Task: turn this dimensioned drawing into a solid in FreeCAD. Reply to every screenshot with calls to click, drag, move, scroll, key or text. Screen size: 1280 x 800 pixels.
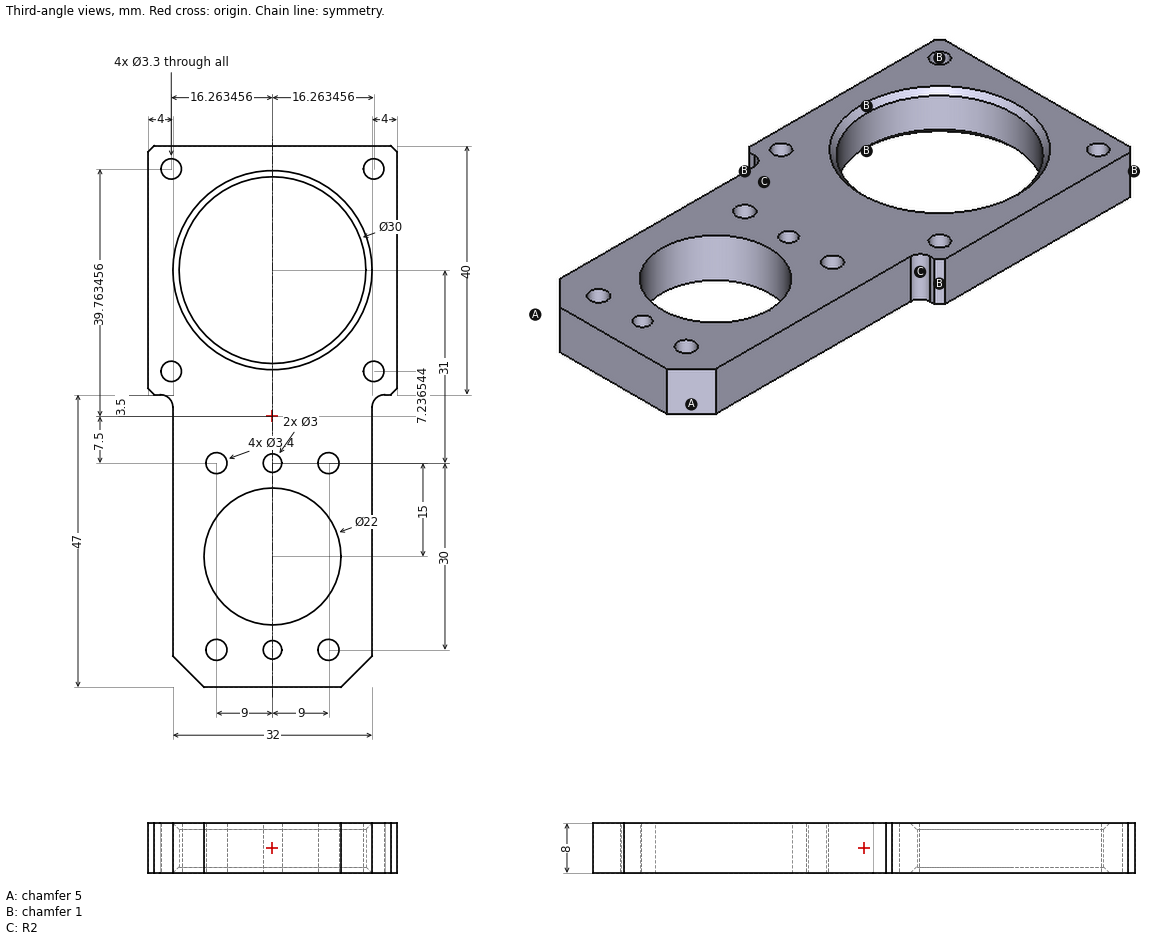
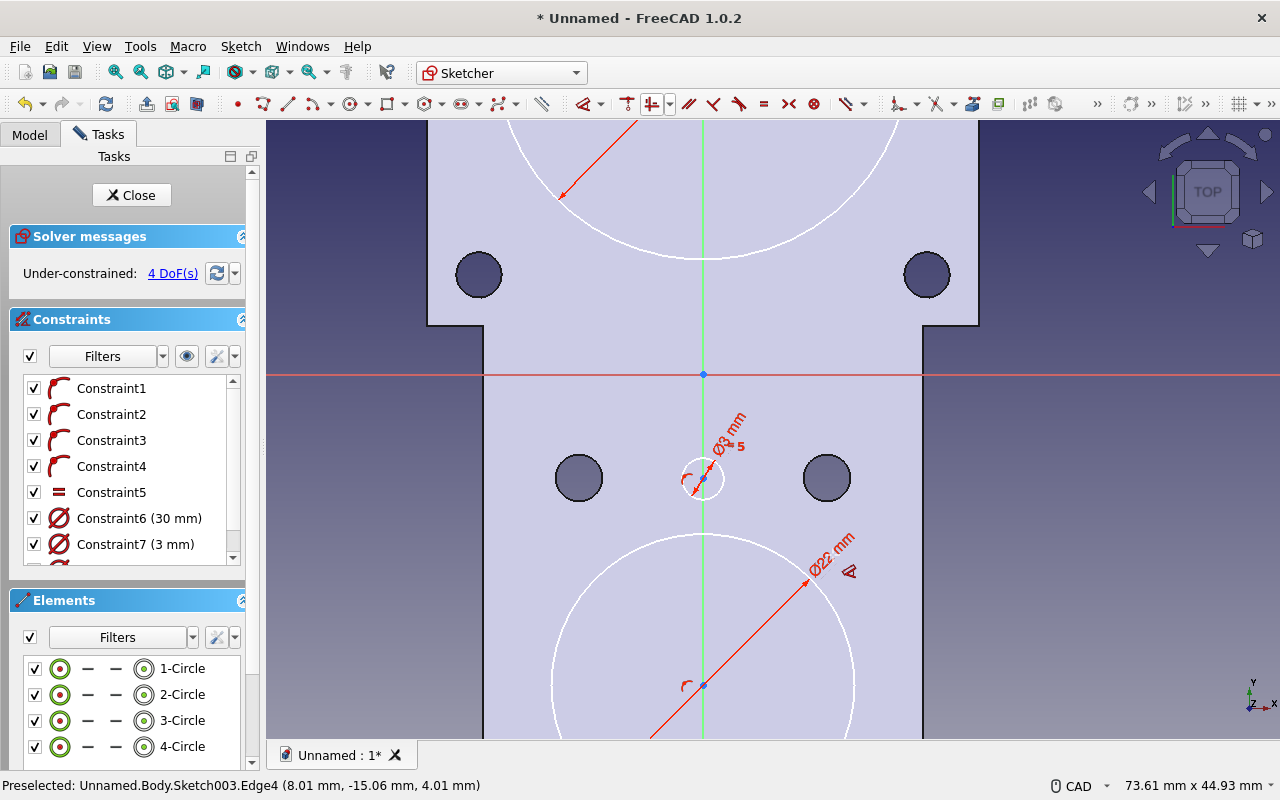
click(703, 479)
click(737, 403)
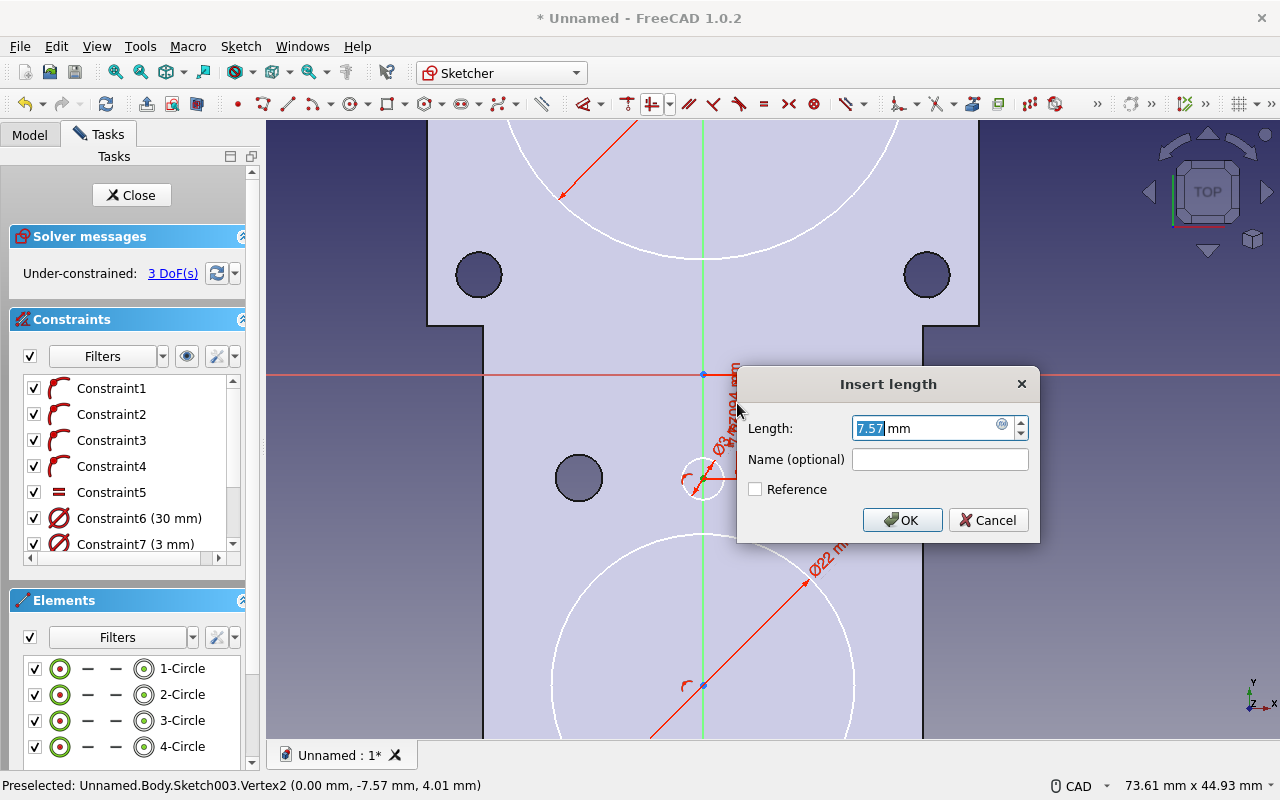
text(7.5)
key(Return)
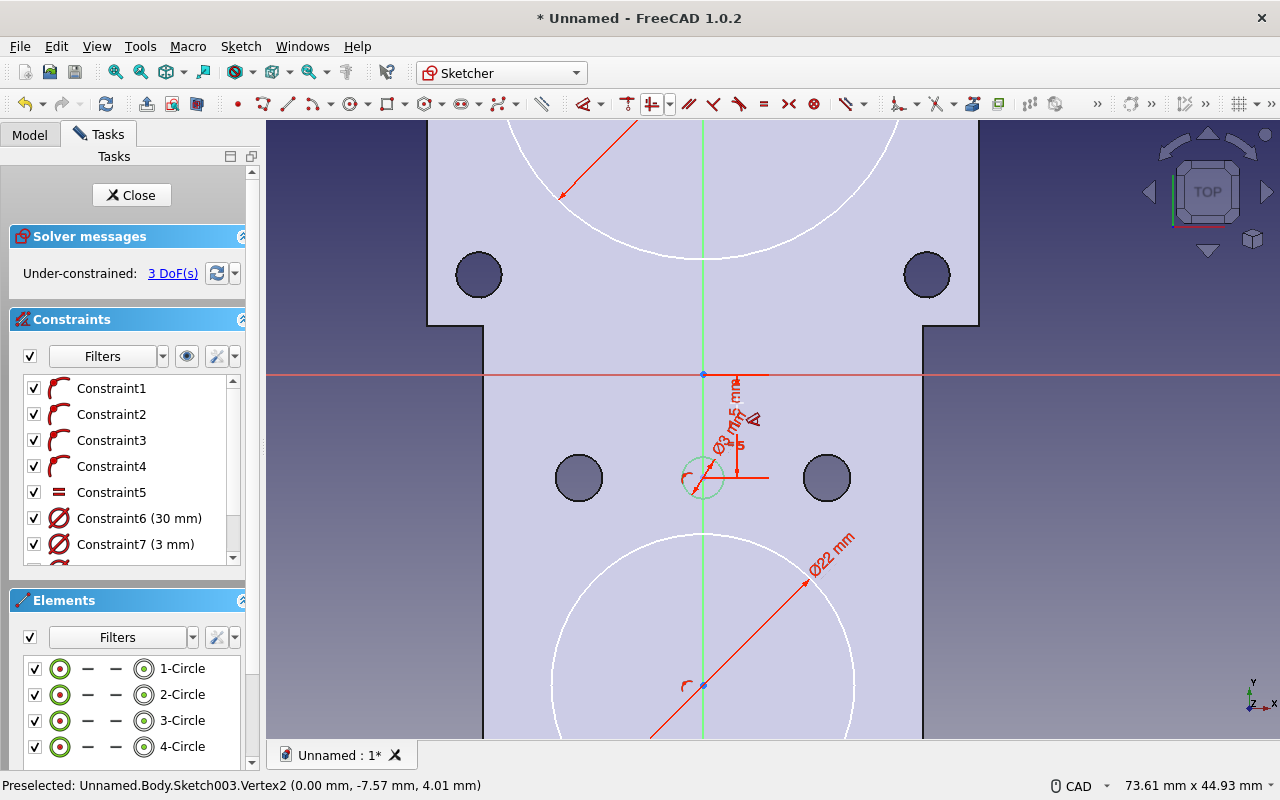
scroll(705, 459, down, 5)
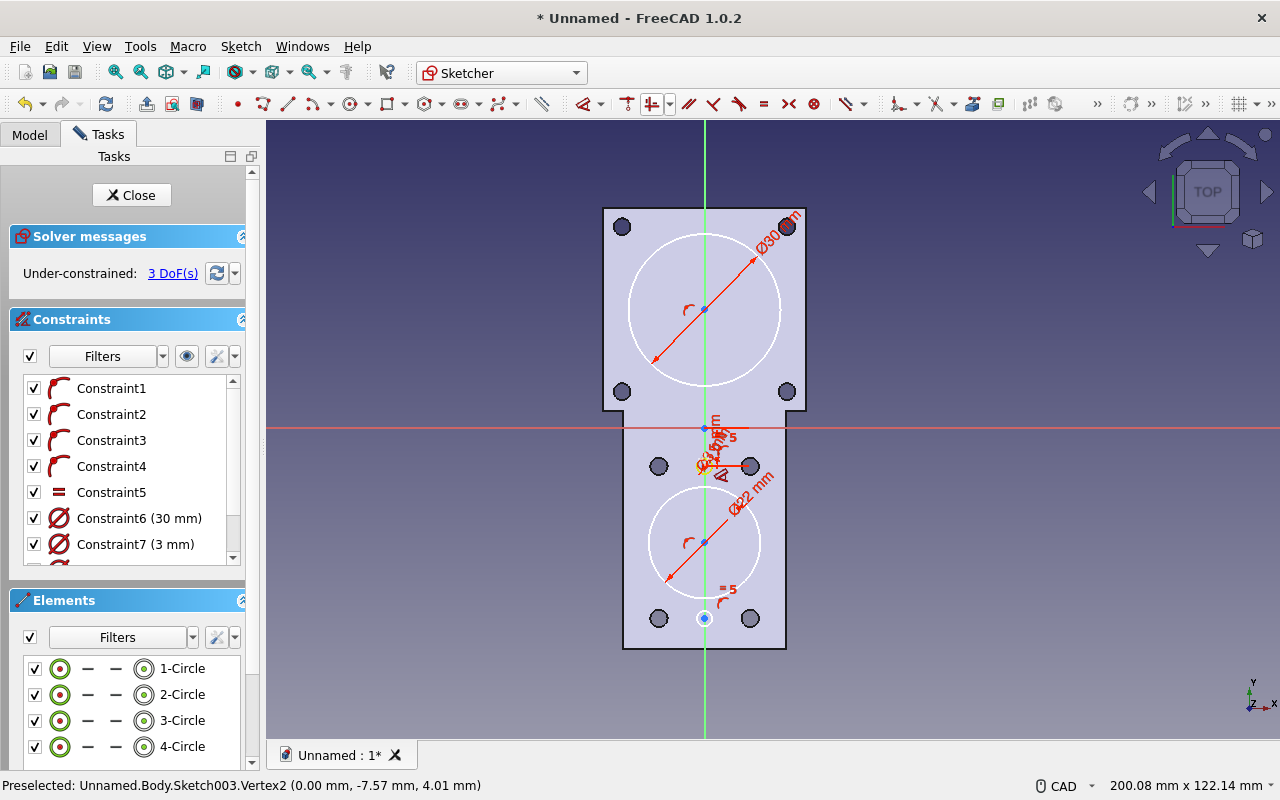
click(705, 310)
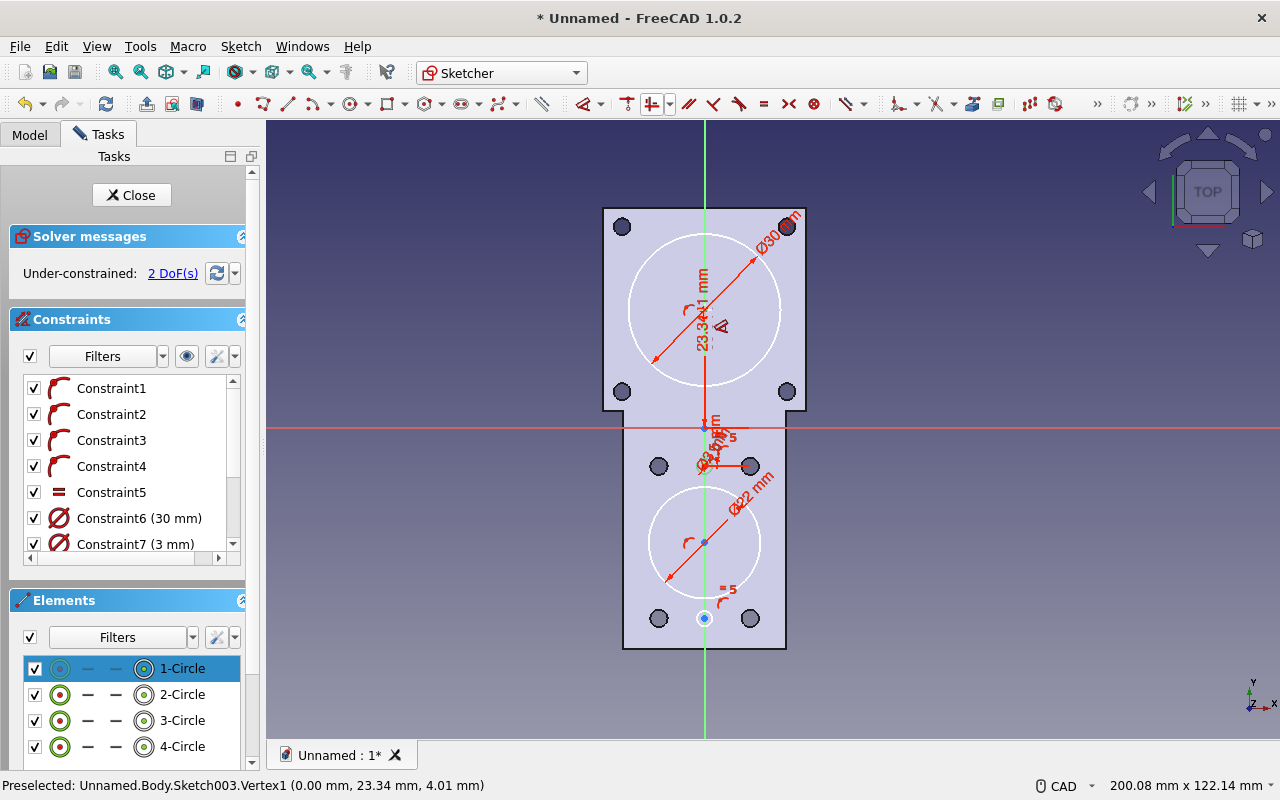
click(705, 466)
click(739, 352)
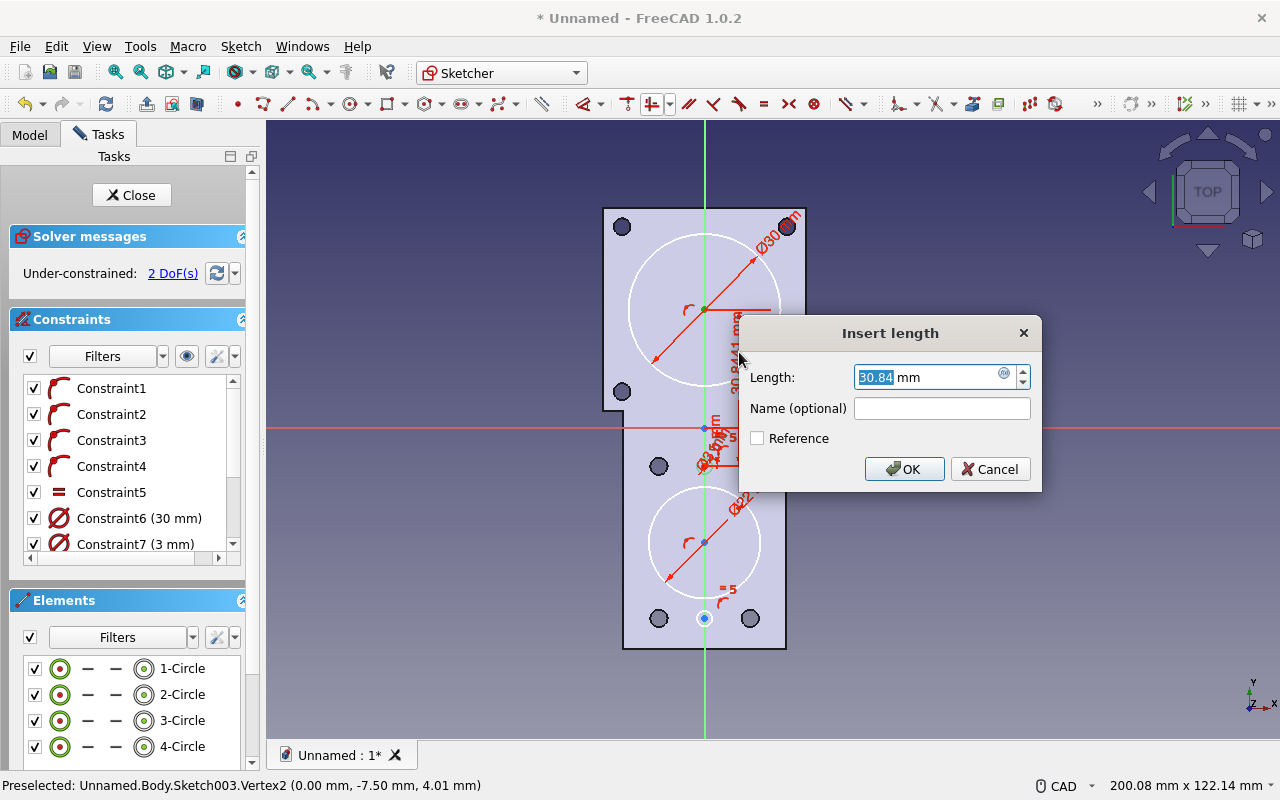
text(31)
key(Return)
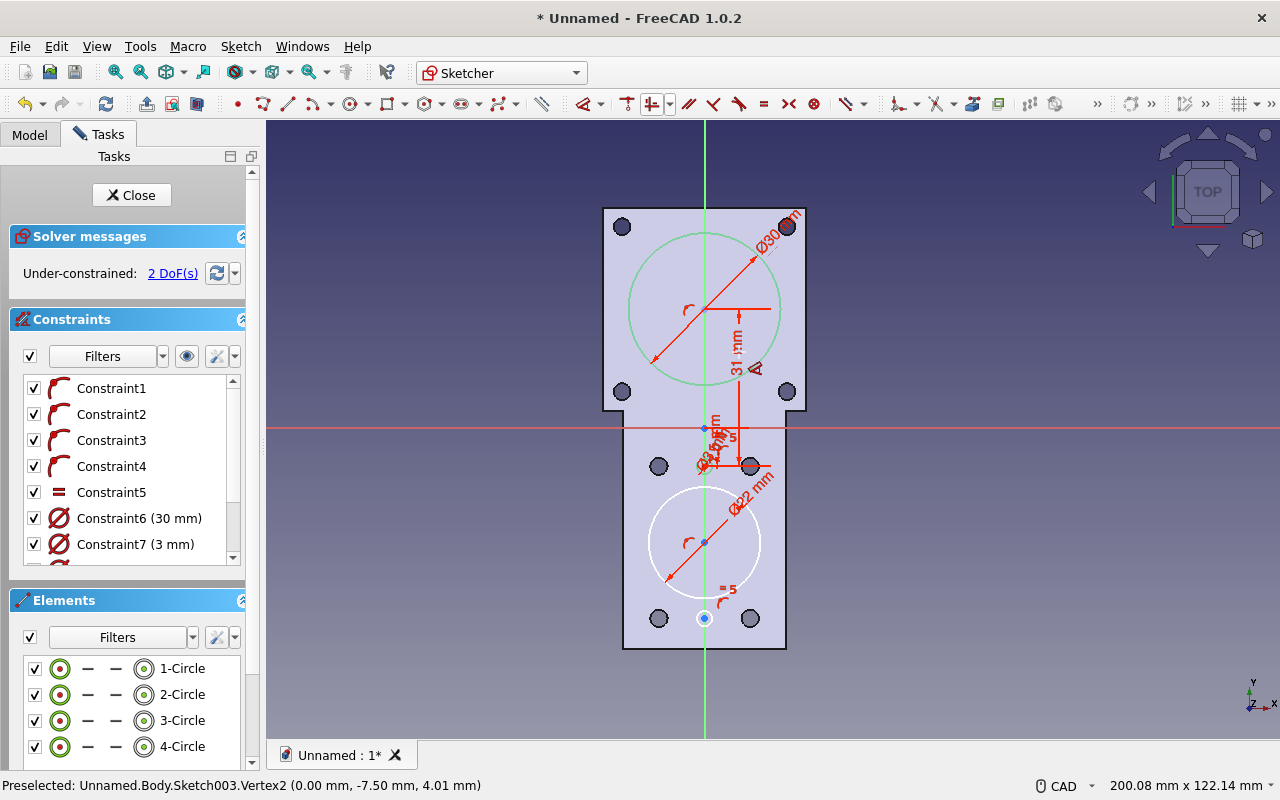
click(705, 466)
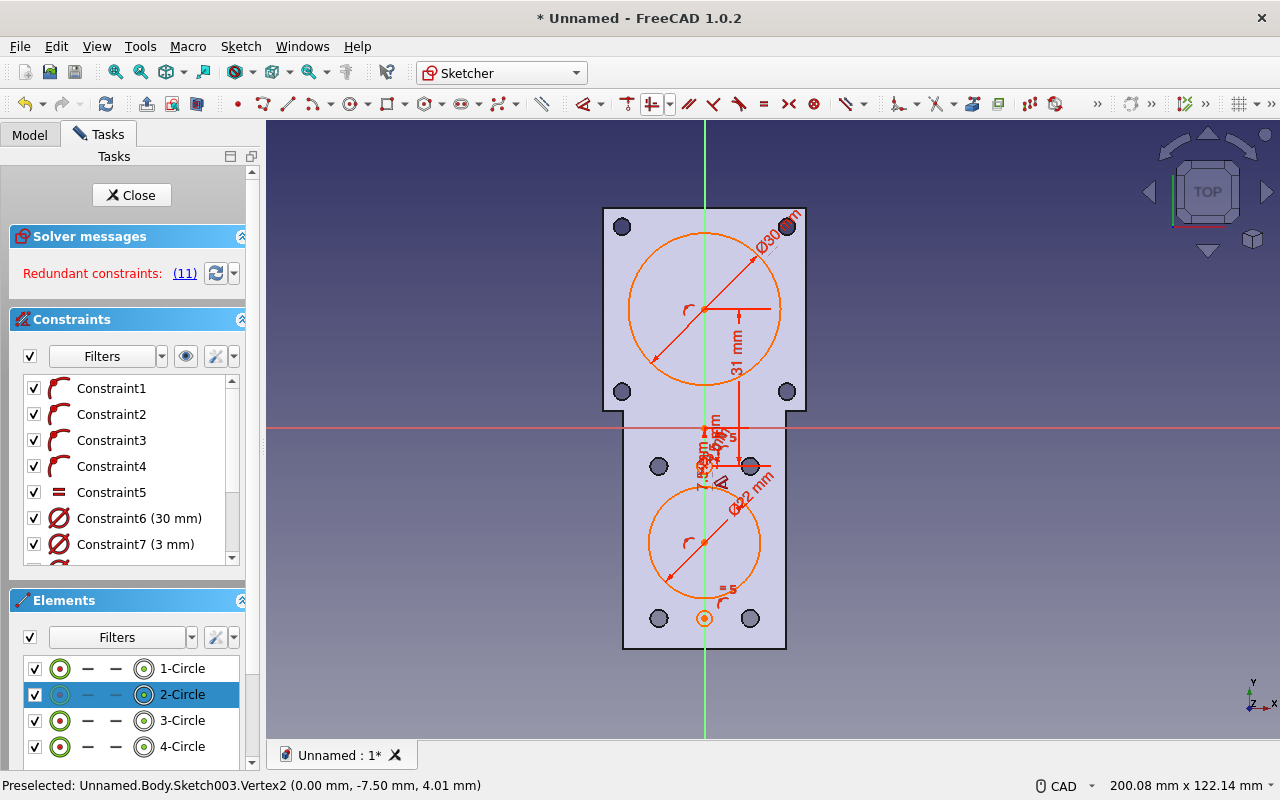
click(705, 619)
click(739, 542)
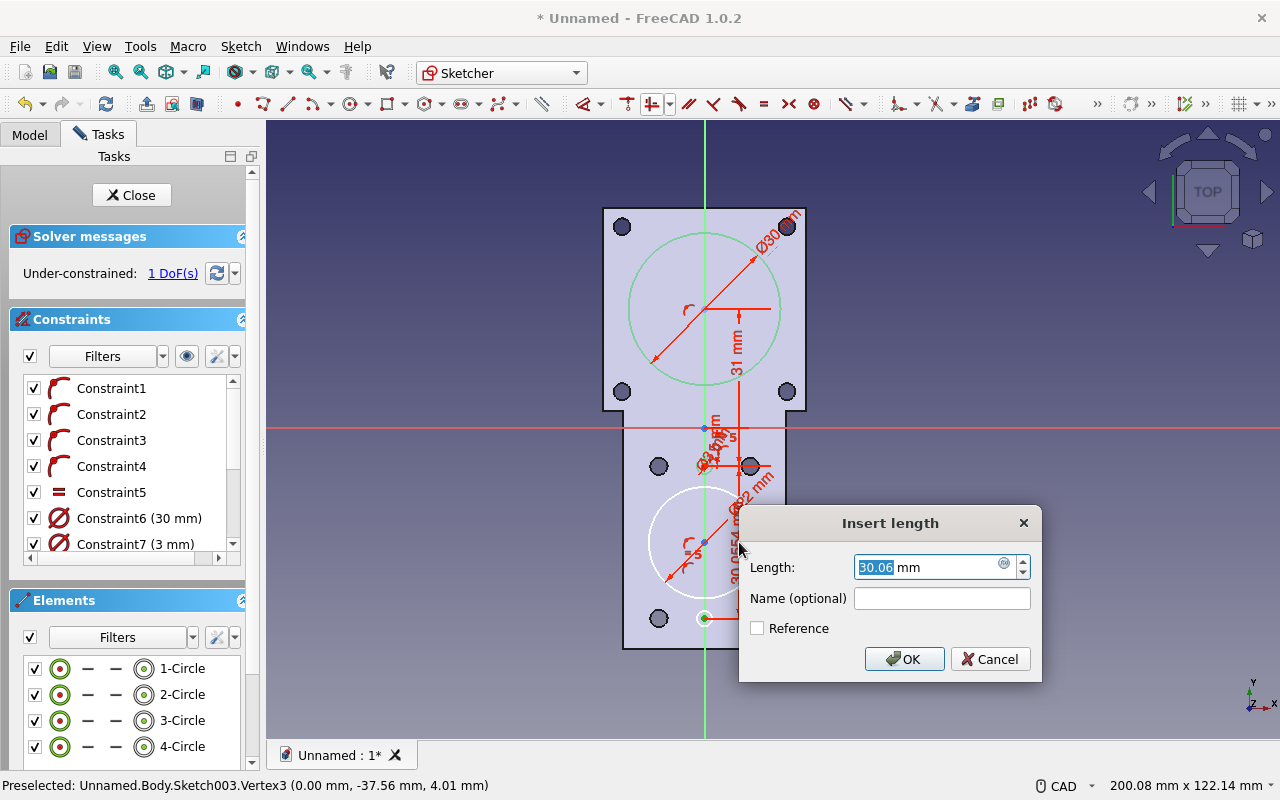
text(30)
key(Return)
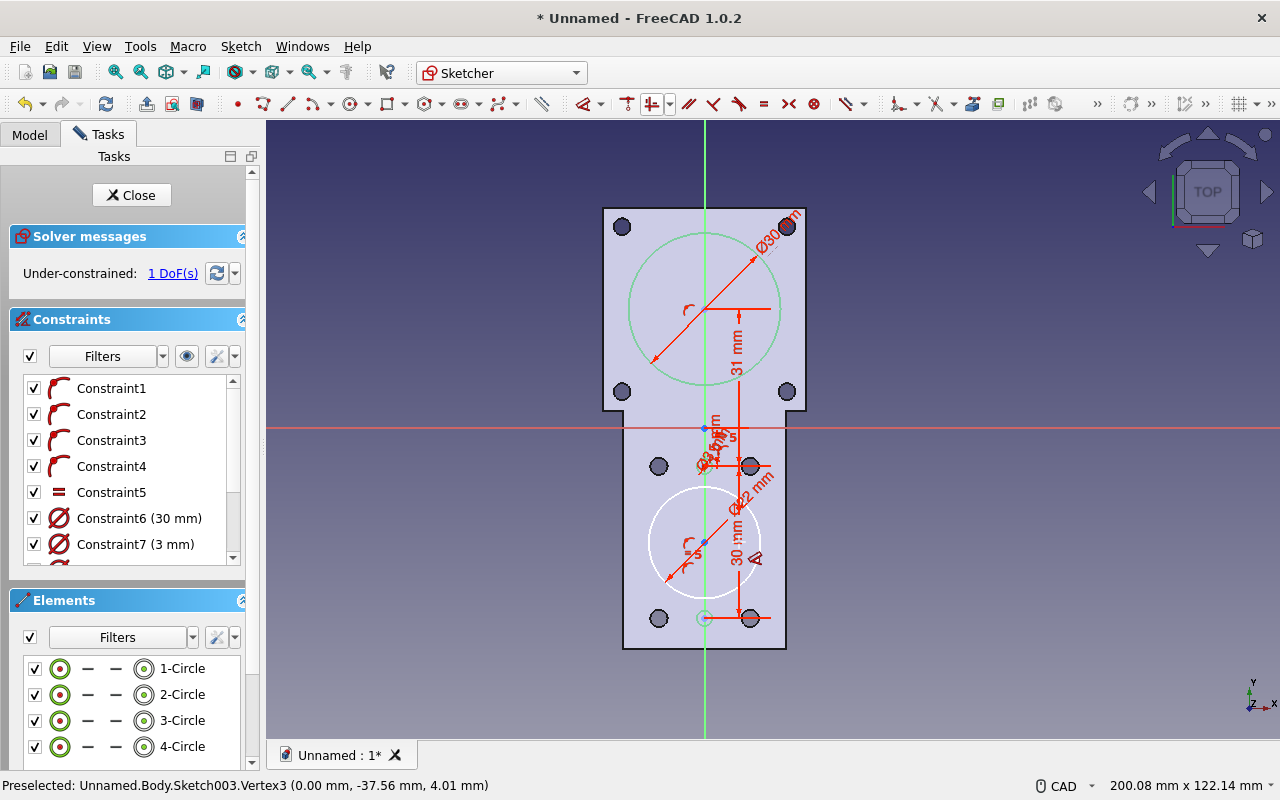
click(705, 466)